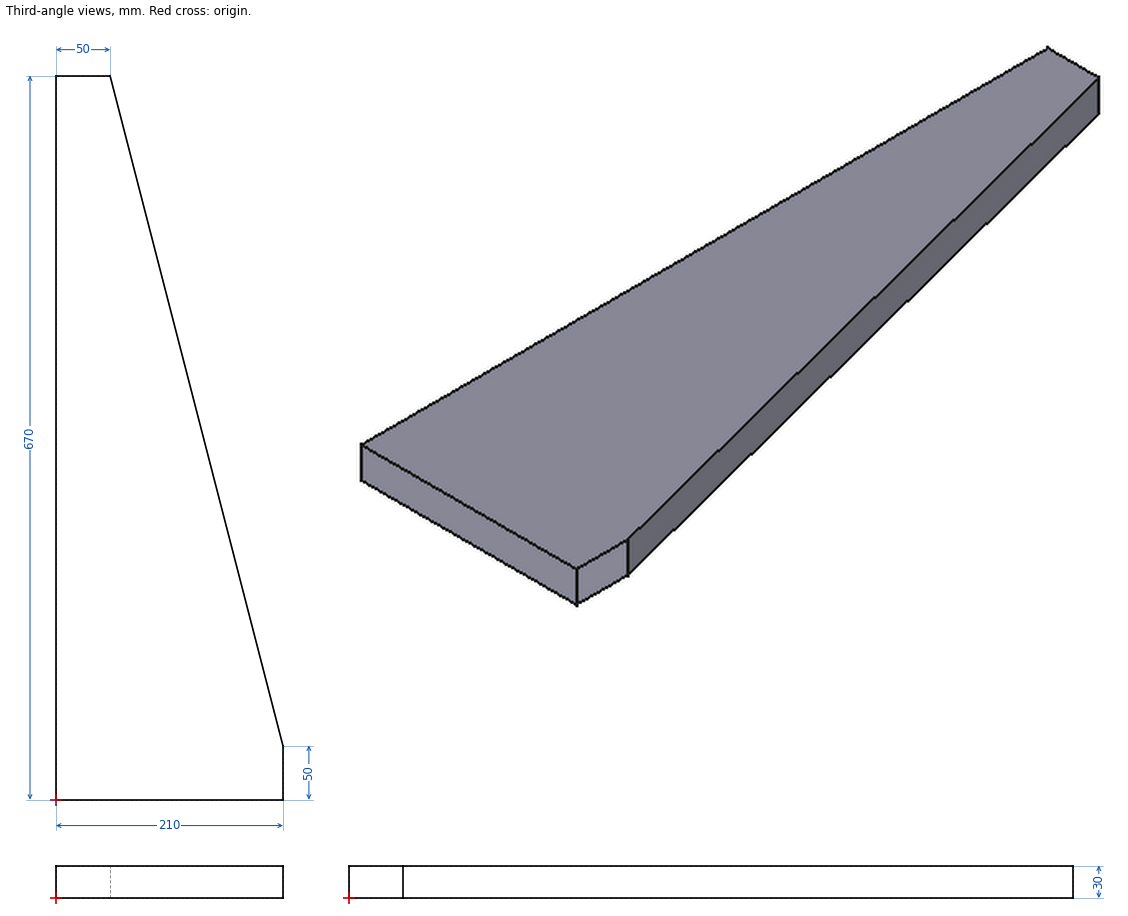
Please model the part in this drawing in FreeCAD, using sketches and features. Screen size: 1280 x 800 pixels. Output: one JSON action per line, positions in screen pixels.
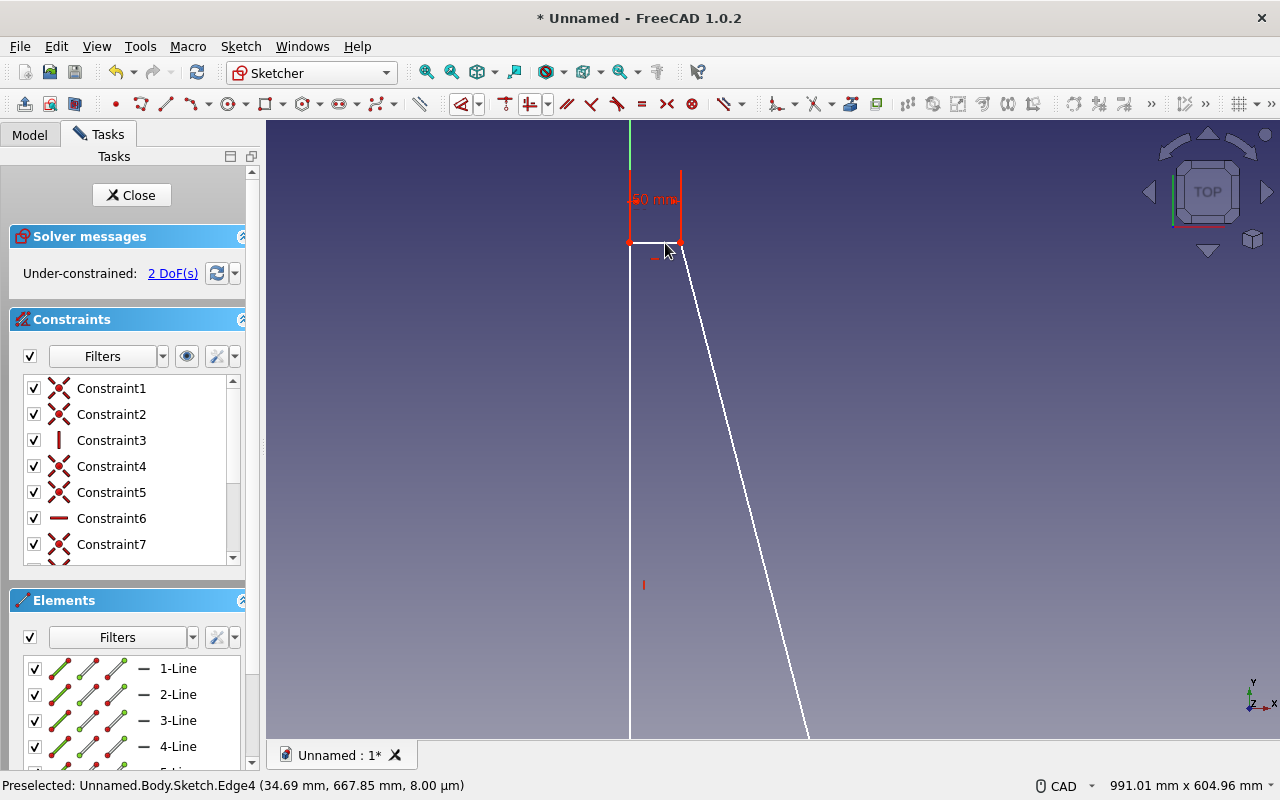
{"action": "scroll", "coordinate": [665, 242], "scroll_direction": "down", "scroll_amount": 3}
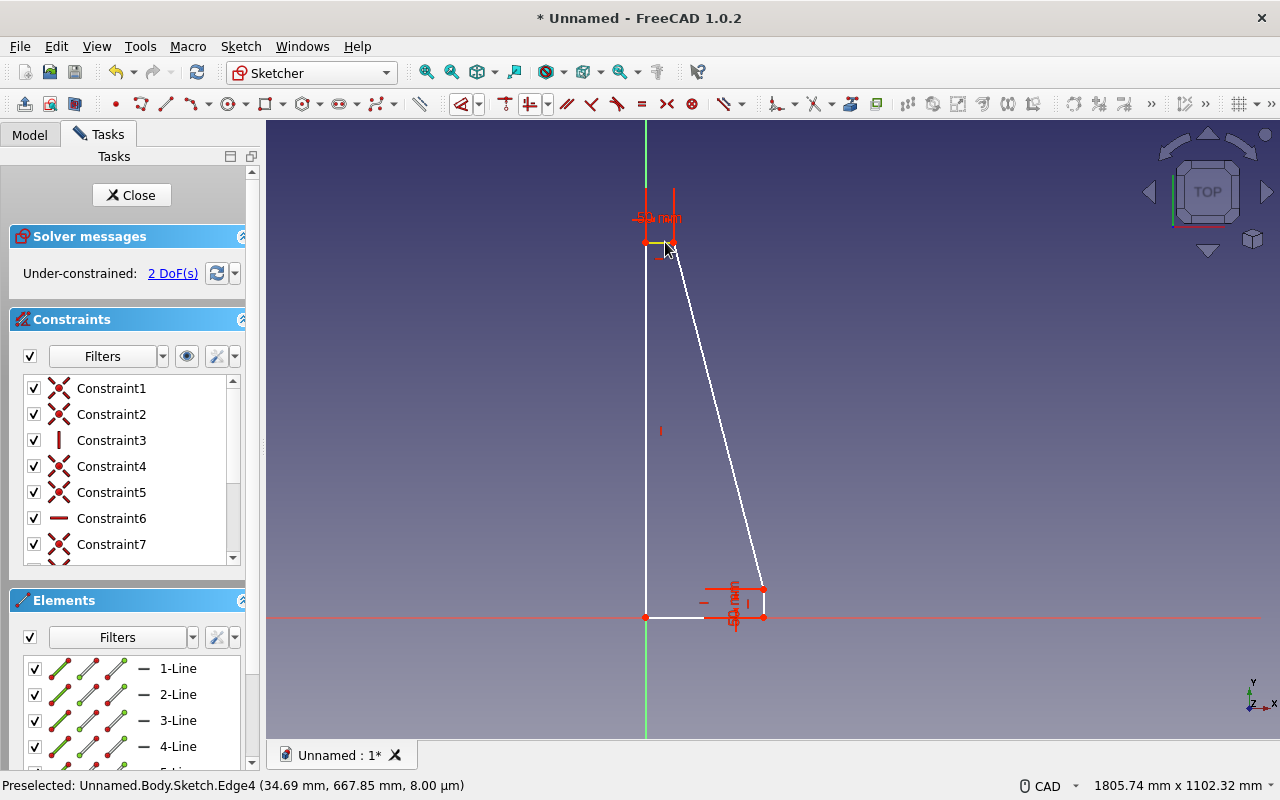
{"action": "left_click", "coordinate": [681, 618]}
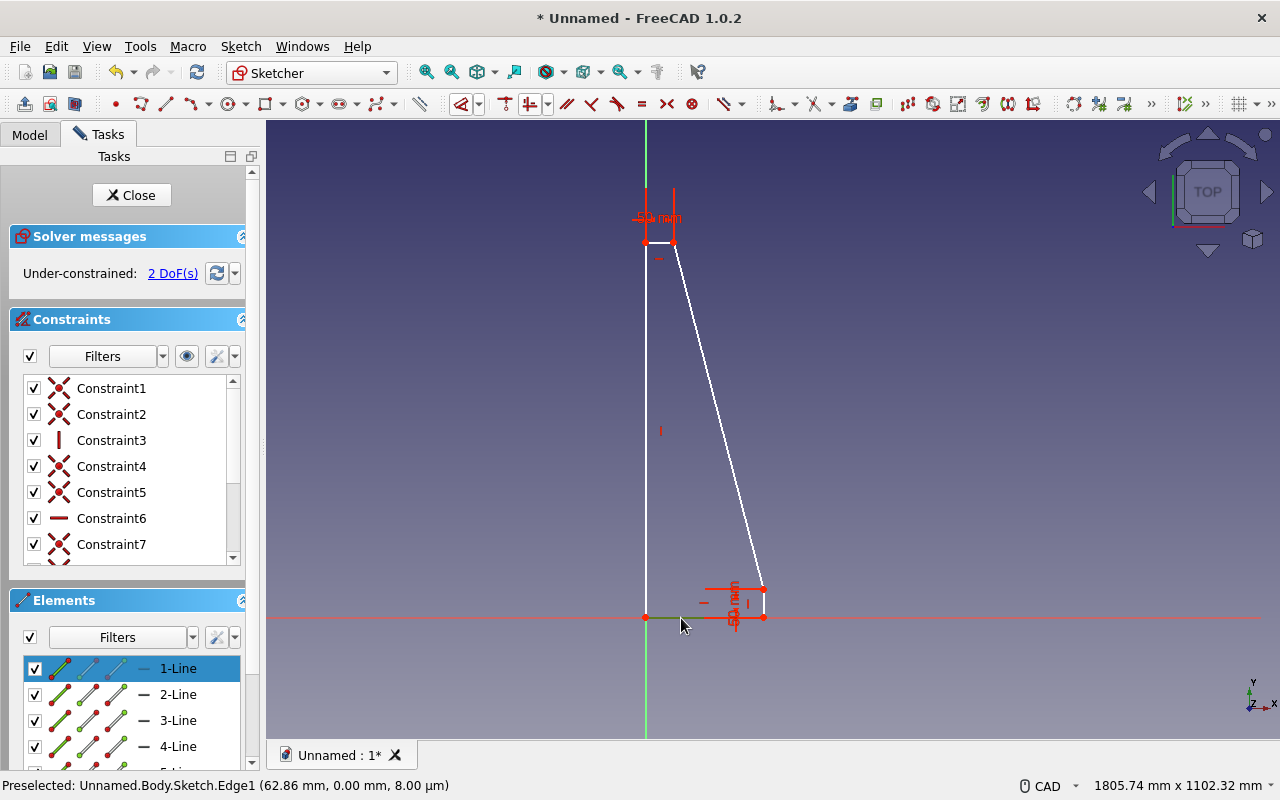
{"action": "key", "text": "l"}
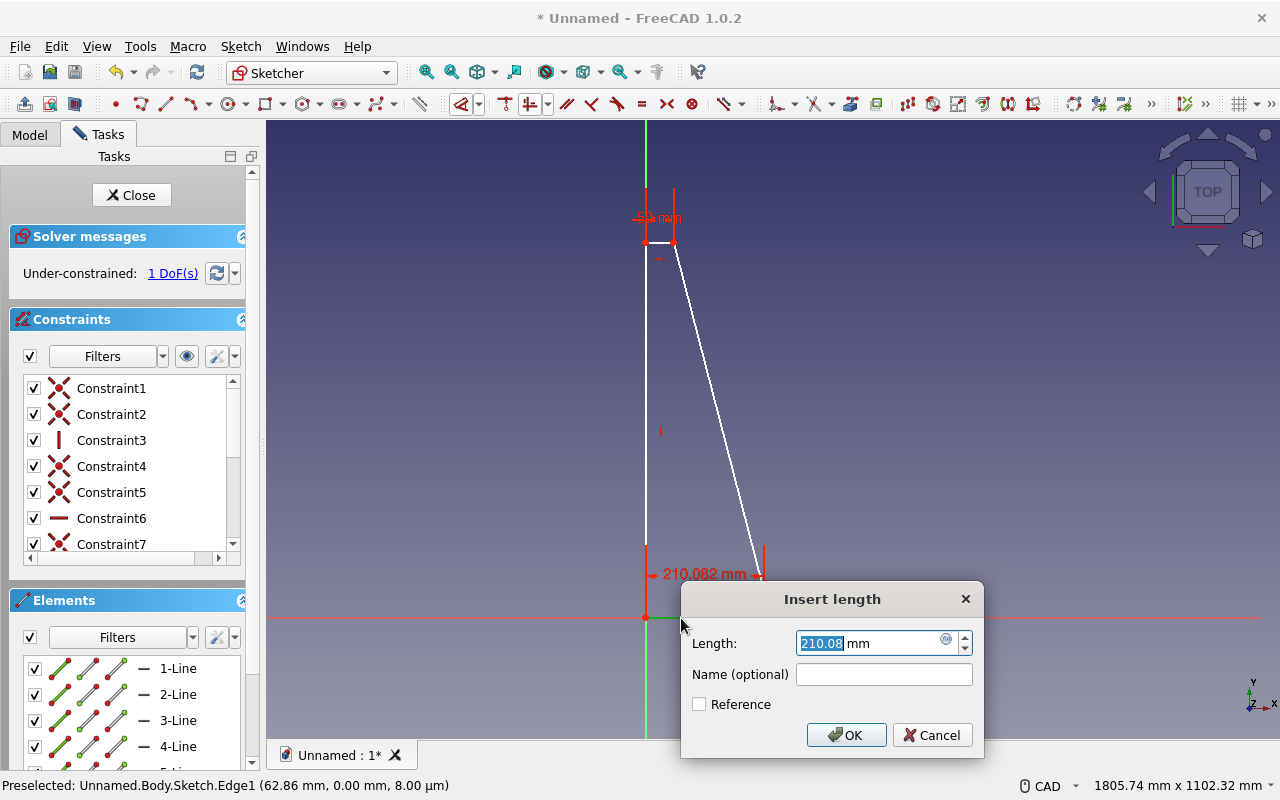
{"action": "type", "text": "210"}
{"action": "key", "text": "Return"}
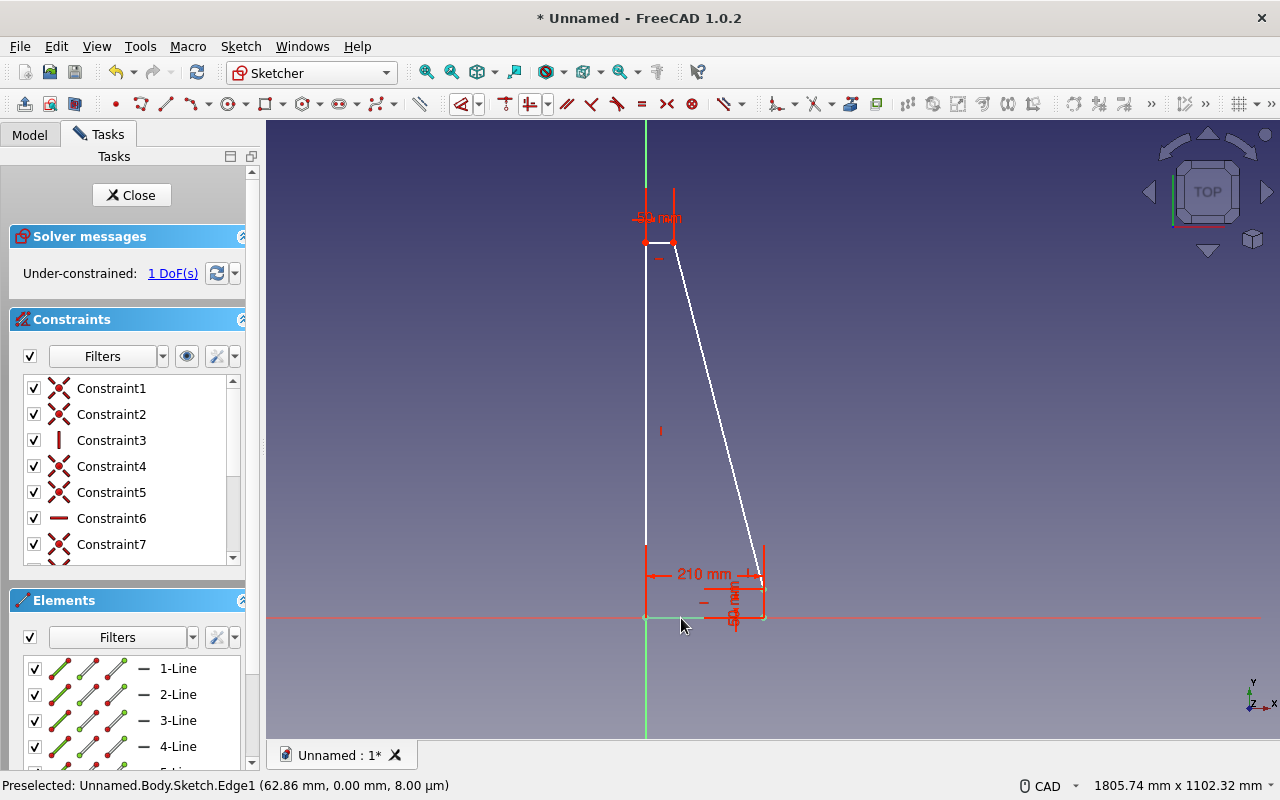
{"action": "left_click", "coordinate": [646, 355]}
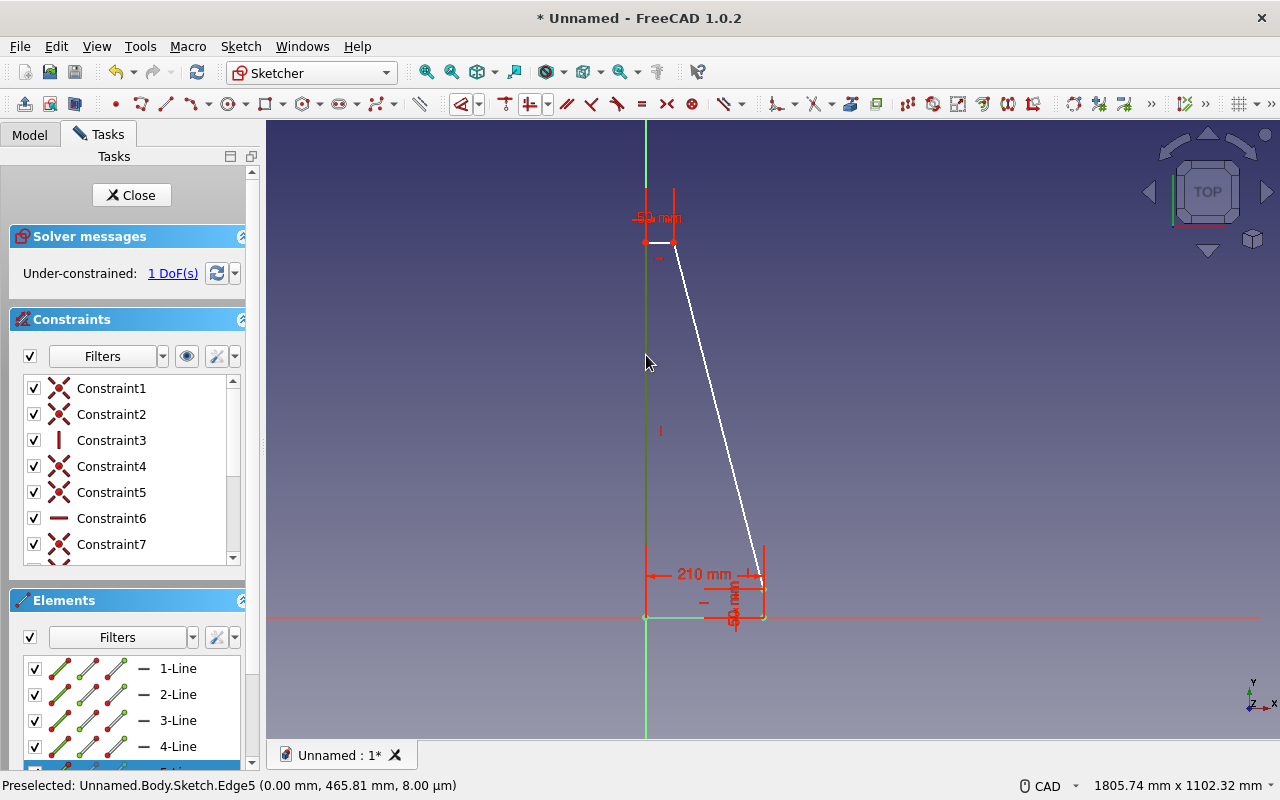
{"action": "left_click", "coordinate": [478, 104]}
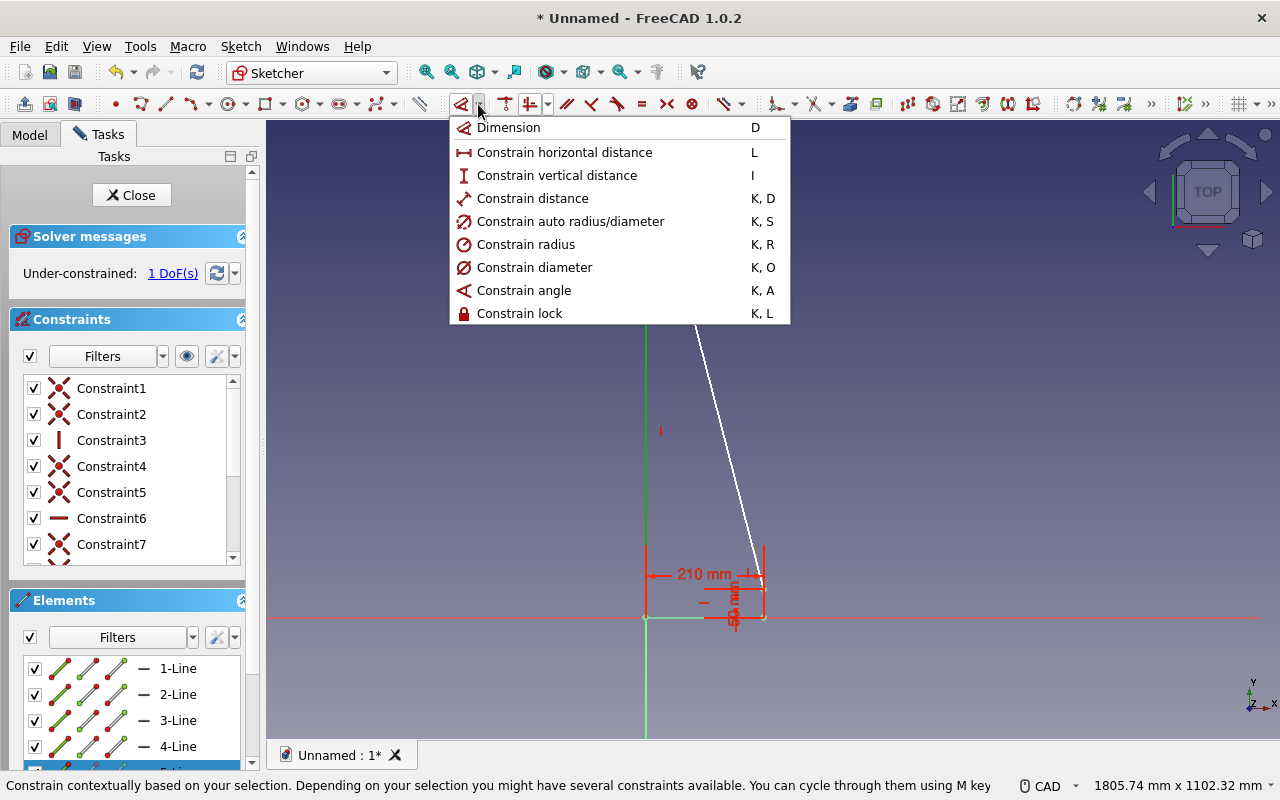
{"action": "left_click", "coordinate": [620, 176]}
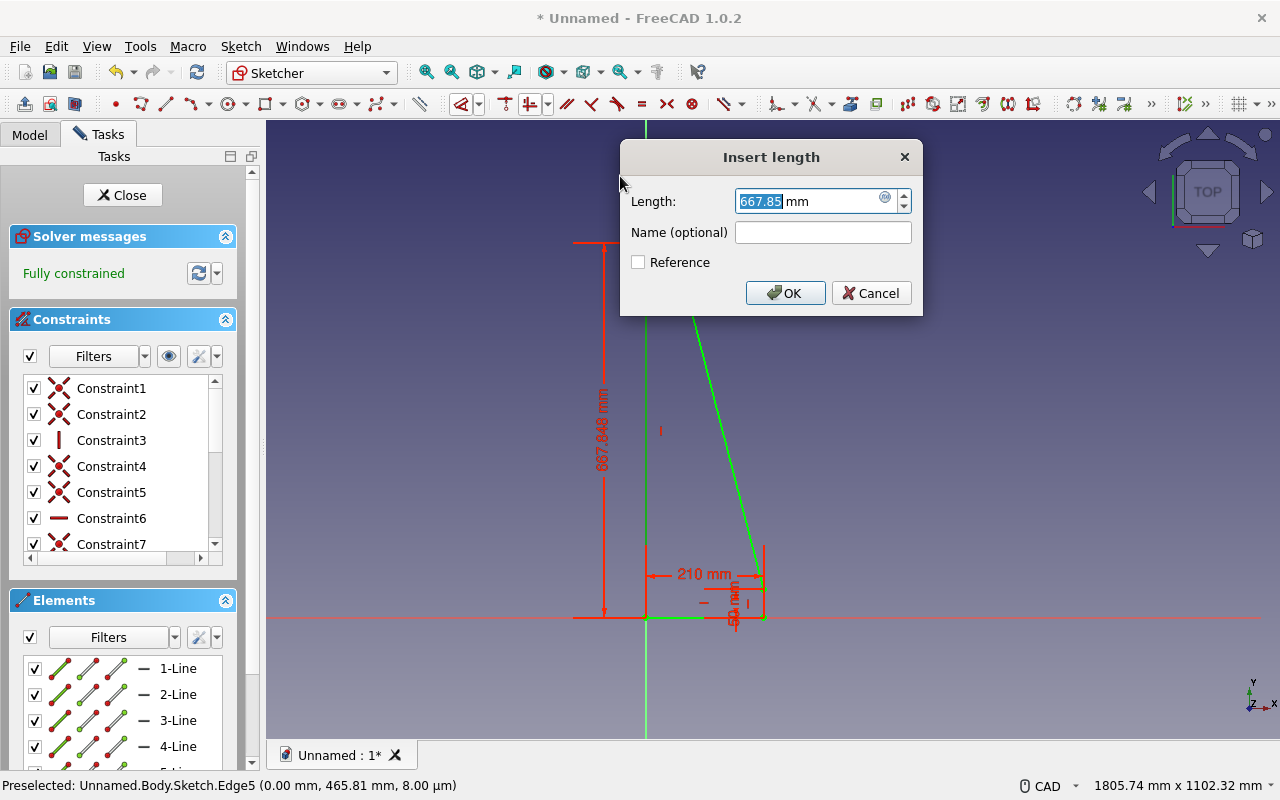
{"action": "type", "text": "670"}
{"action": "key", "text": "Return"}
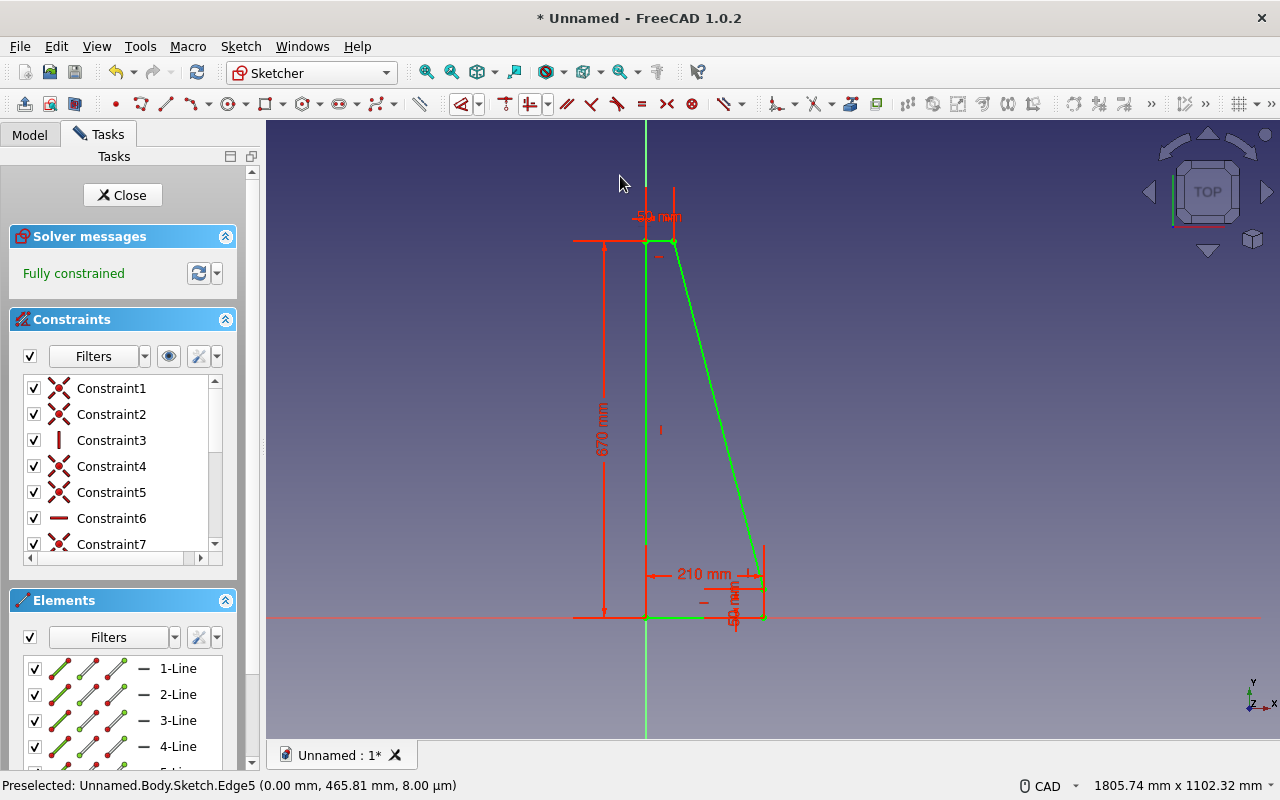
{"action": "left_click", "coordinate": [123, 195]}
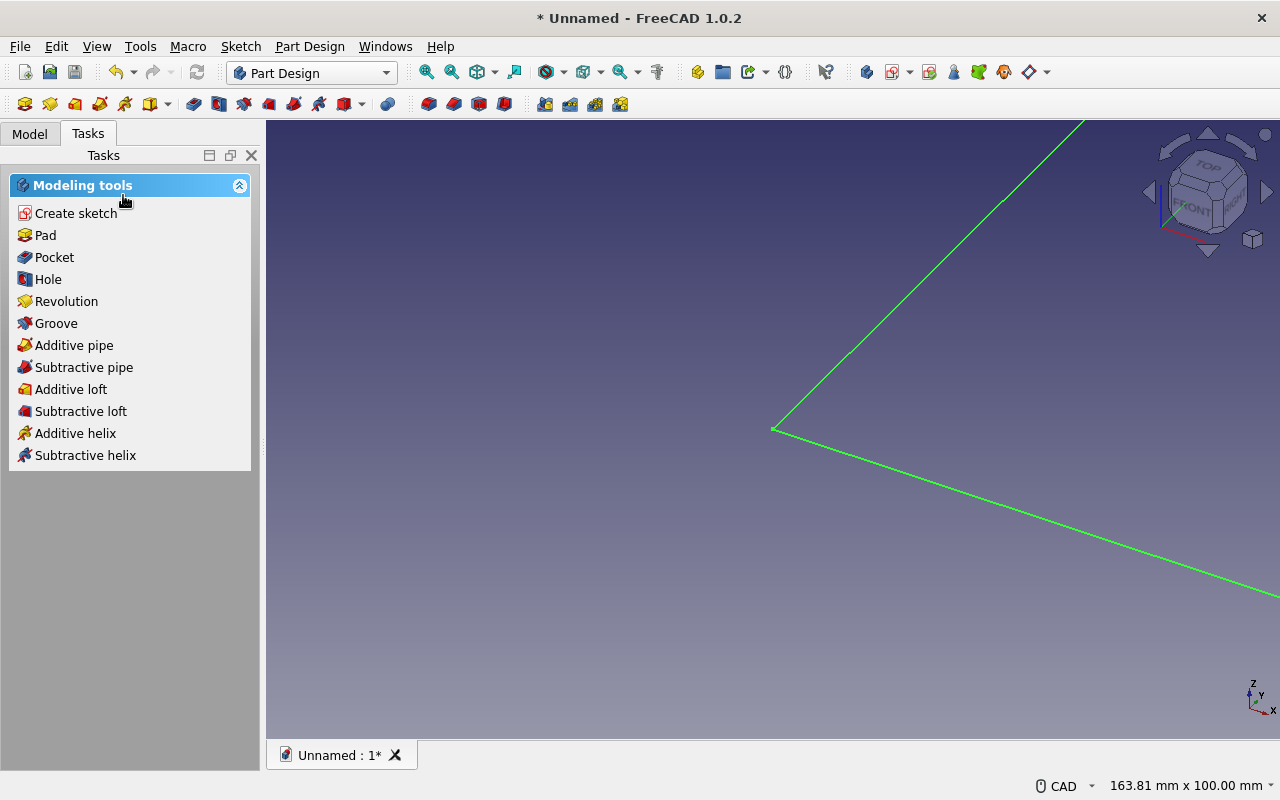
{"action": "left_click", "coordinate": [25, 104]}